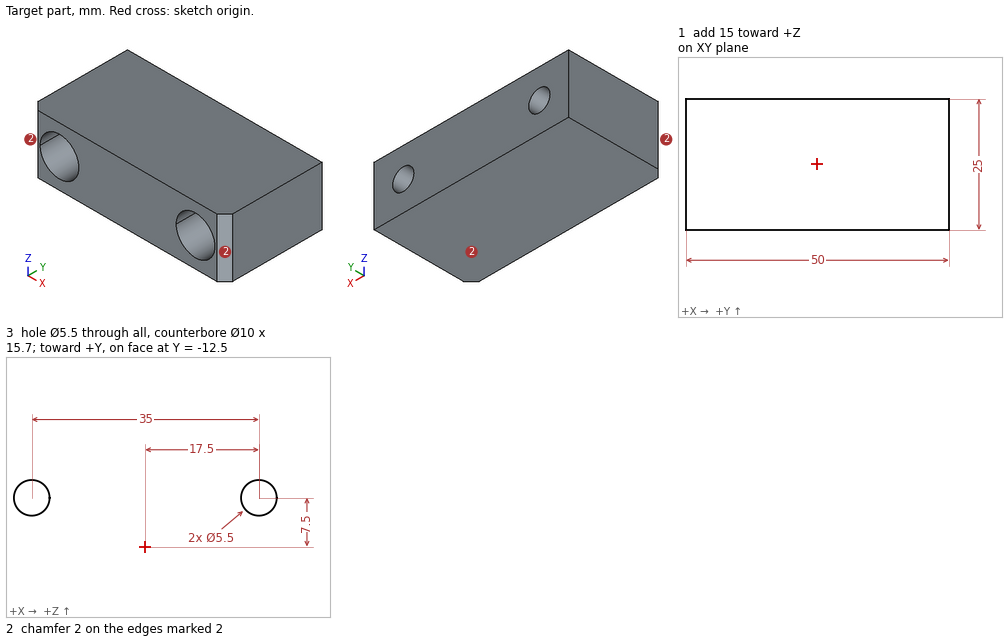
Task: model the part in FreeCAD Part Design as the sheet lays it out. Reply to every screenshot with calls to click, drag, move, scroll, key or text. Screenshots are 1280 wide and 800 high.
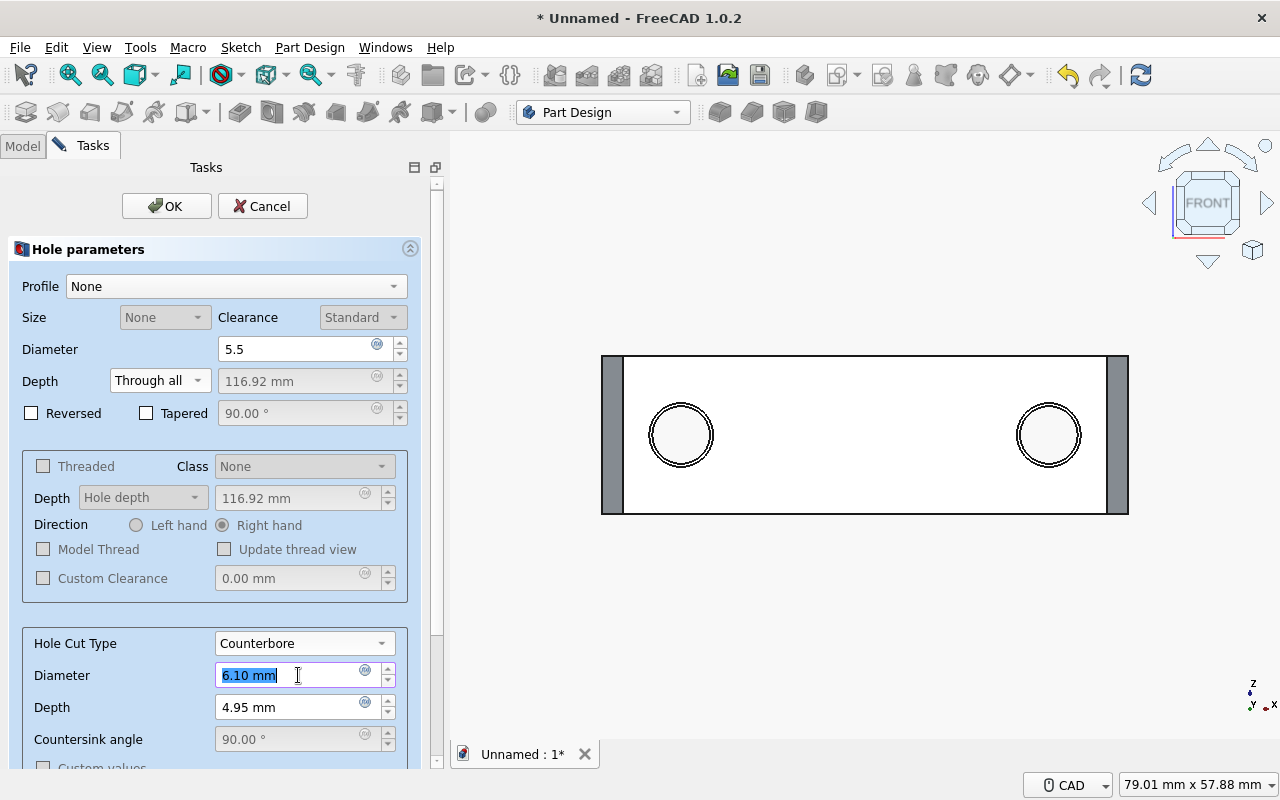
text(10)
key(Tab)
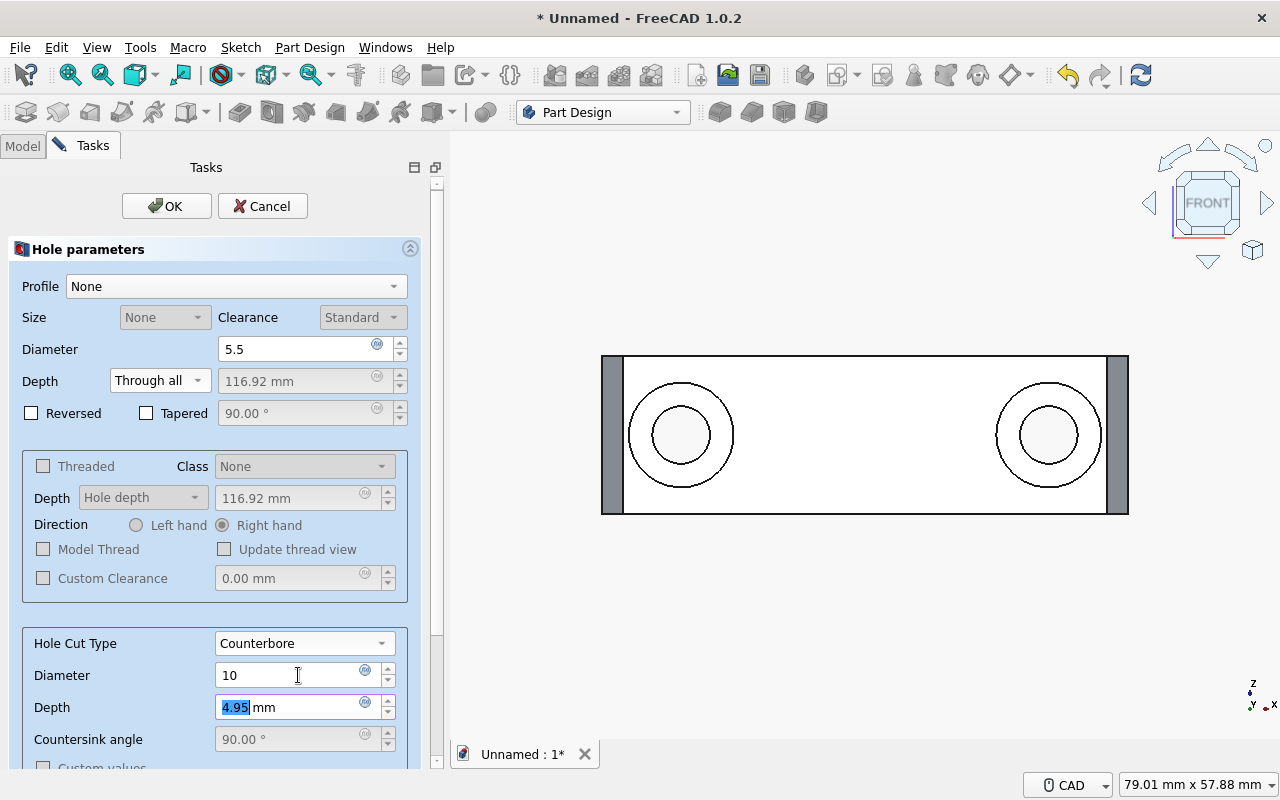
text(15.7)
key(Tab)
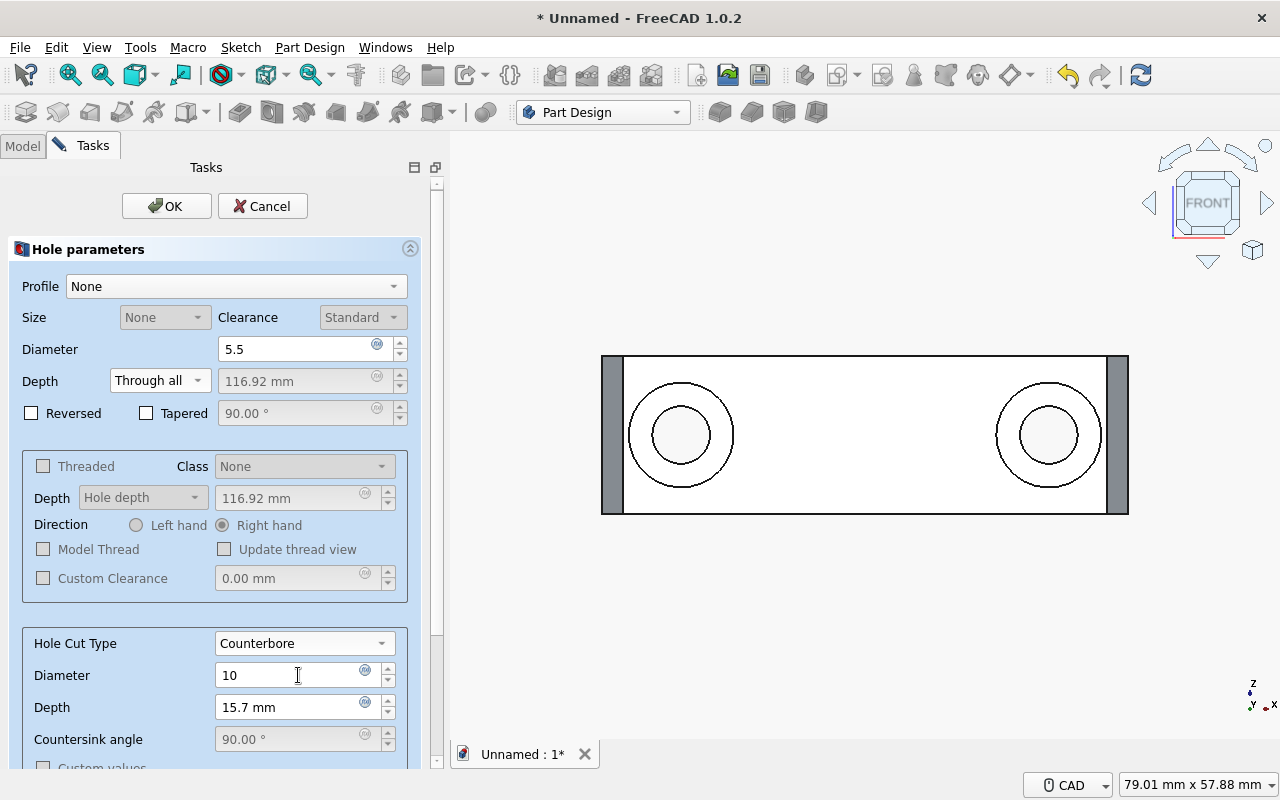
click(167, 206)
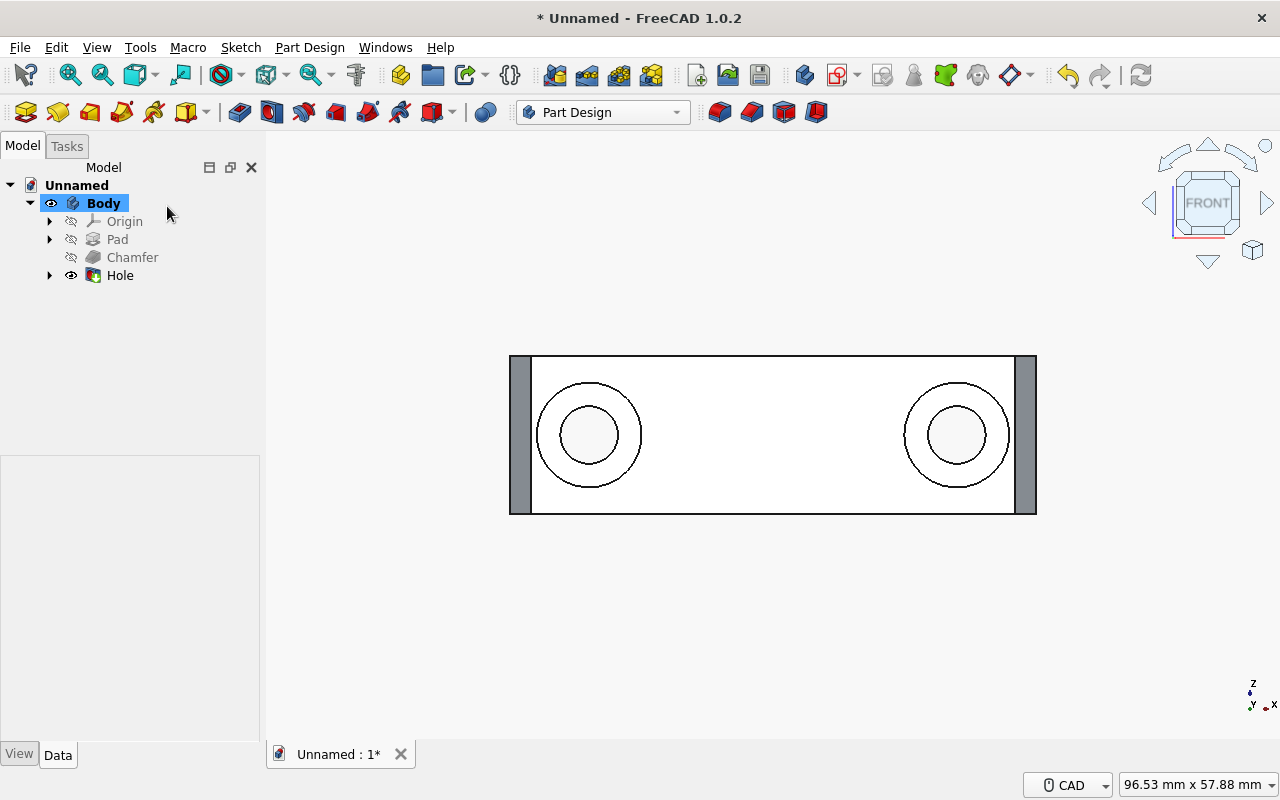
key(0)